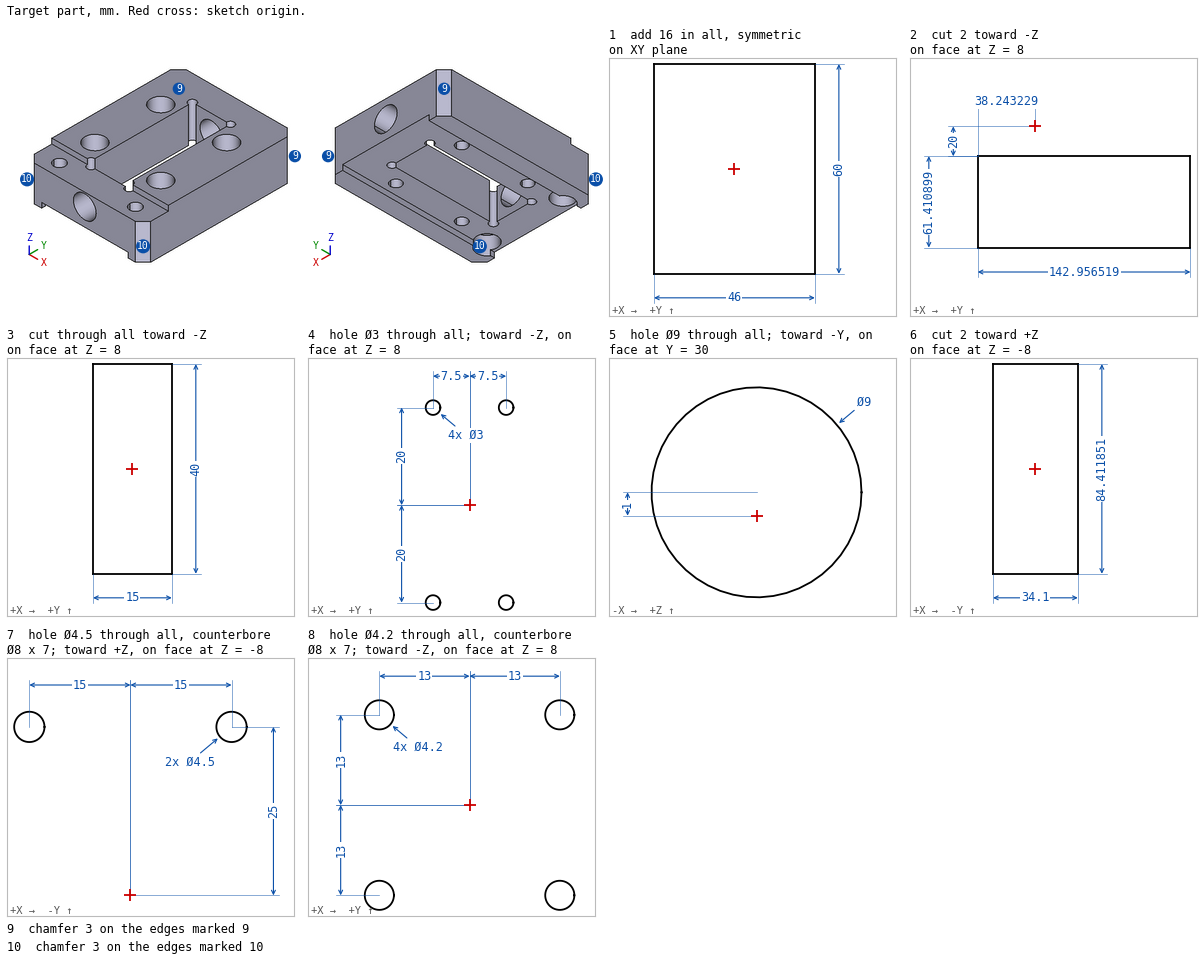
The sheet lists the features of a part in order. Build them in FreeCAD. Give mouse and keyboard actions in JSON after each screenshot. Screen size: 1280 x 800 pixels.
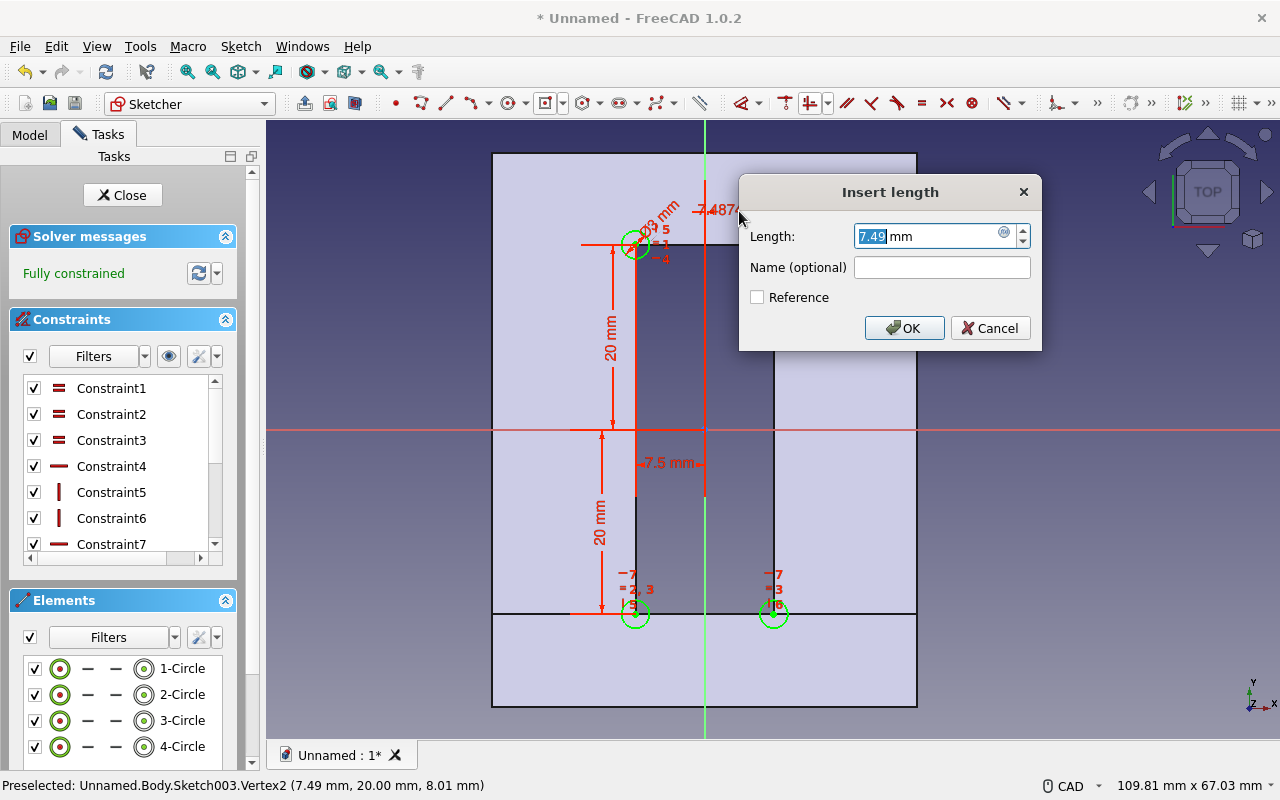
{"action": "type", "text": "7.5"}
{"action": "key", "text": "Return"}
{"action": "key", "text": "Escape"}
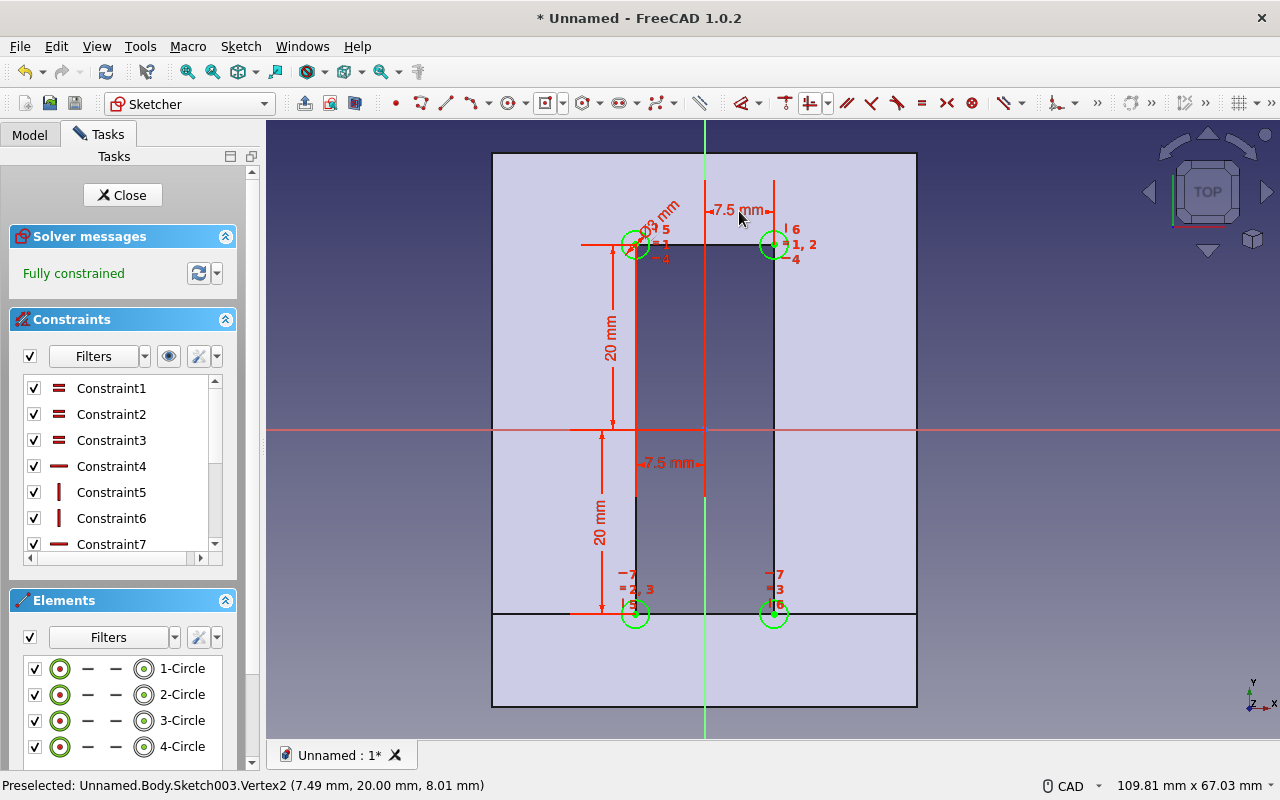
{"action": "left_click", "coordinate": [123, 195]}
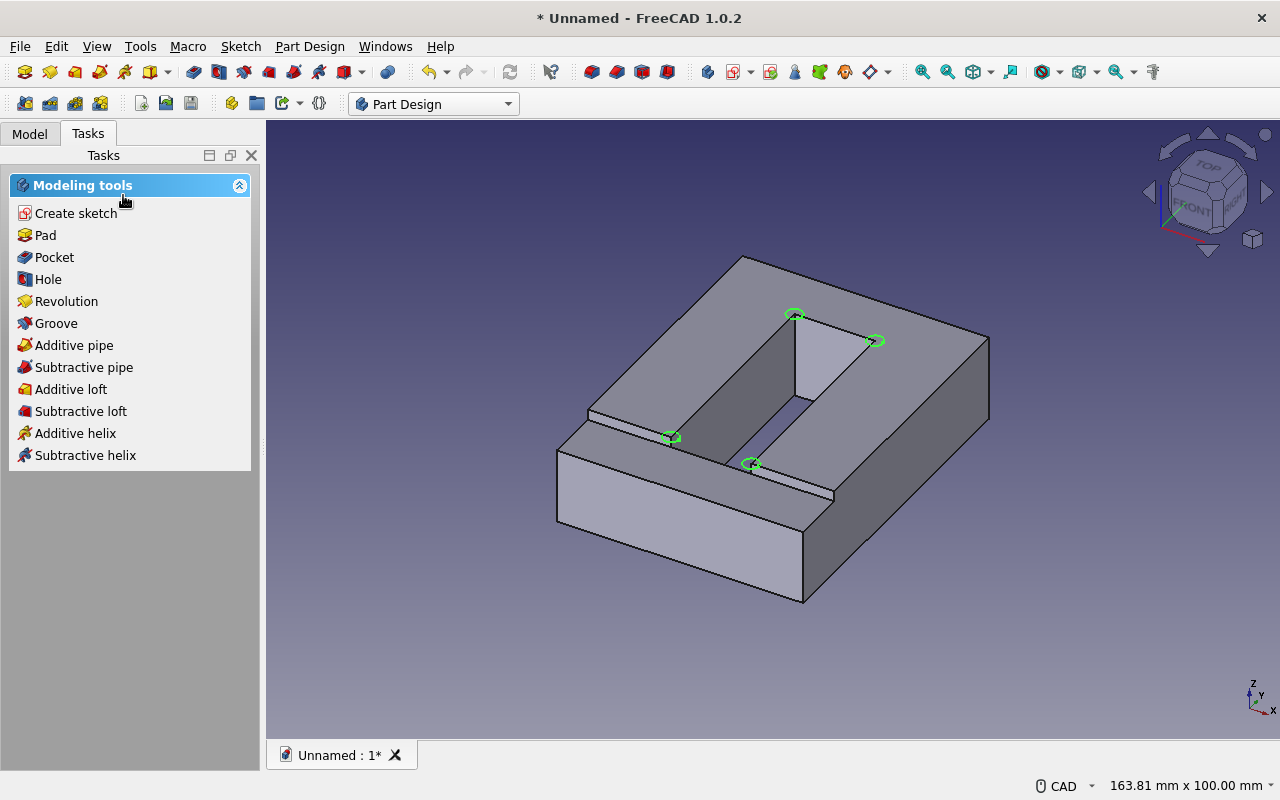
{"action": "left_click", "coordinate": [219, 72]}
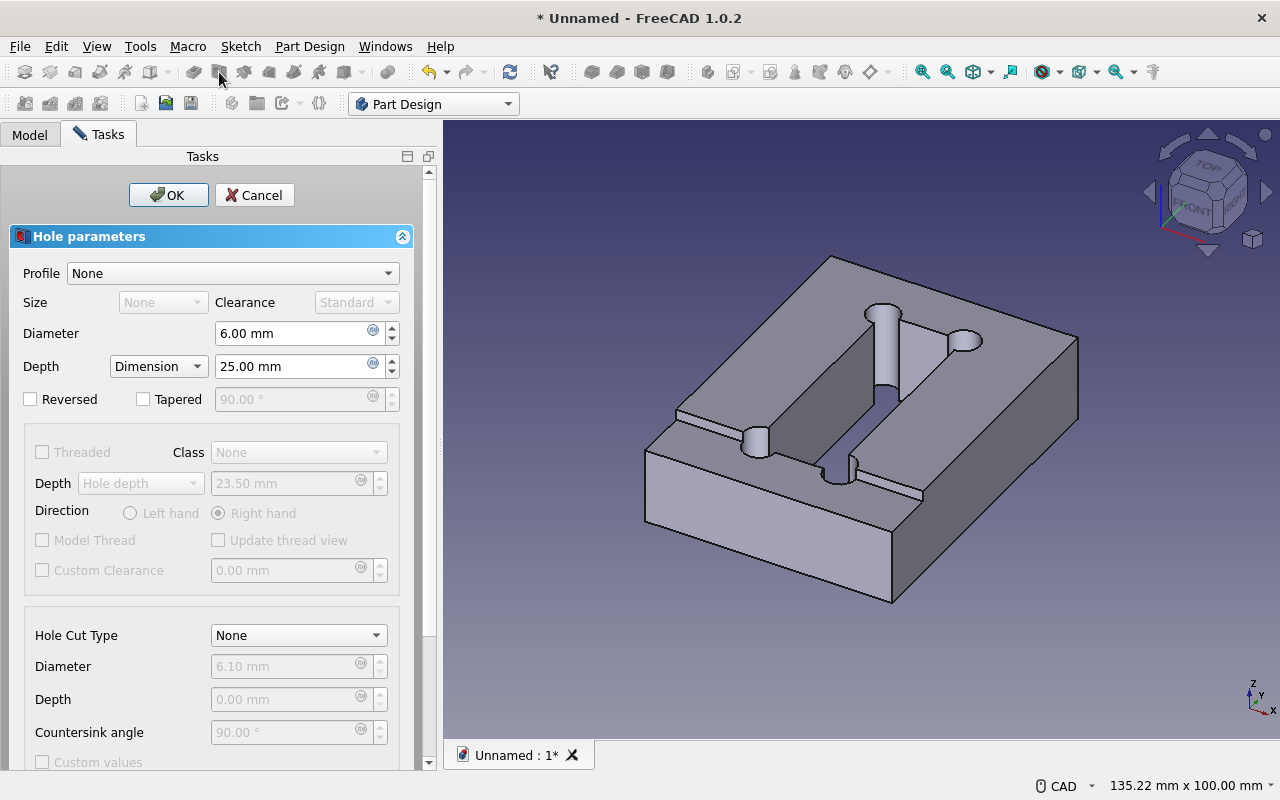
{"action": "triple_click", "coordinate": [300, 334]}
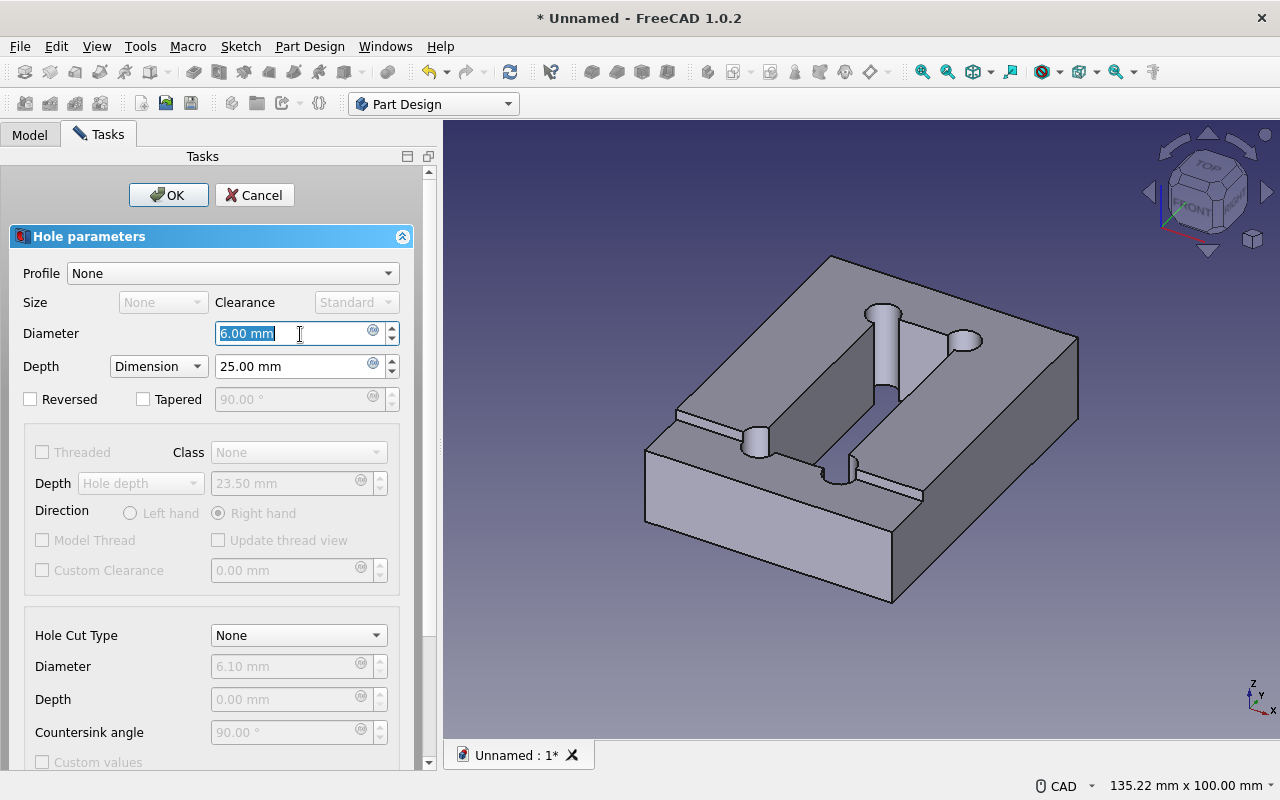
{"action": "type", "text": "3"}
{"action": "key", "text": "Tab"}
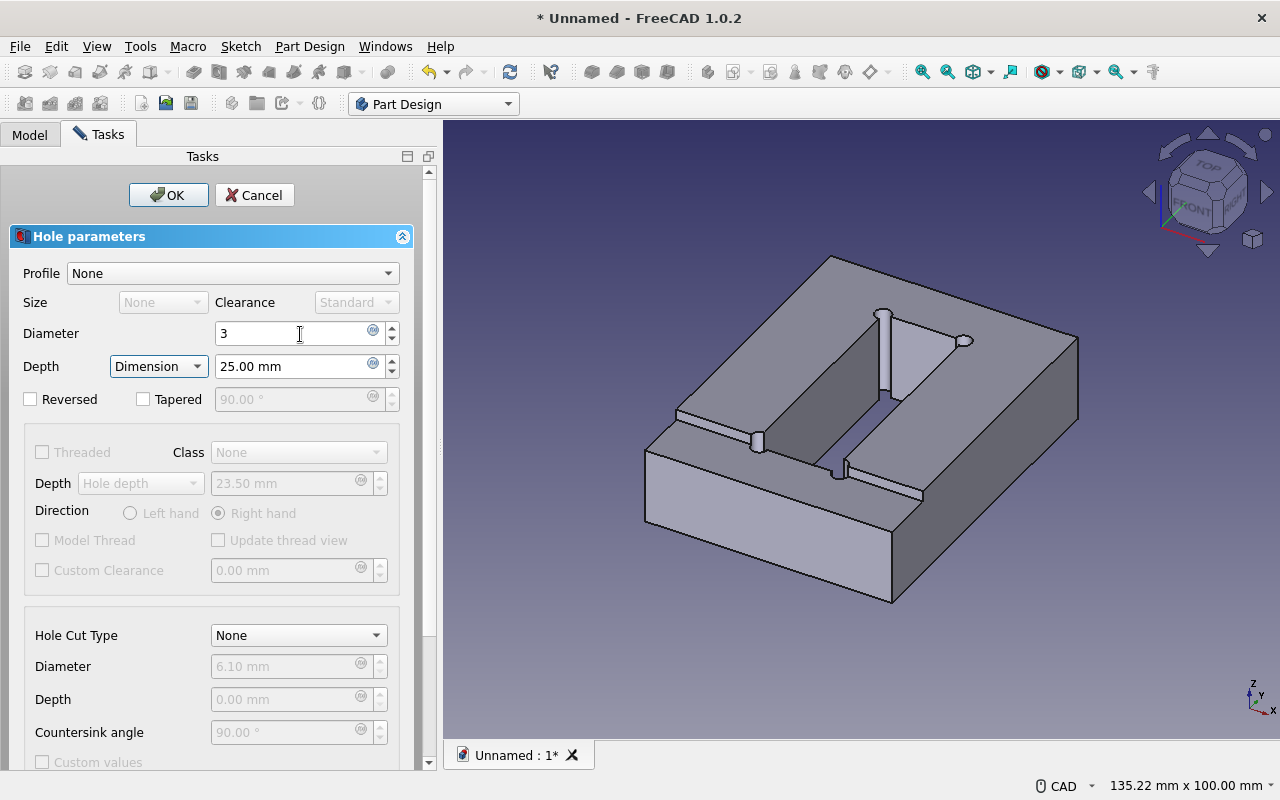
{"action": "left_click", "coordinate": [160, 366]}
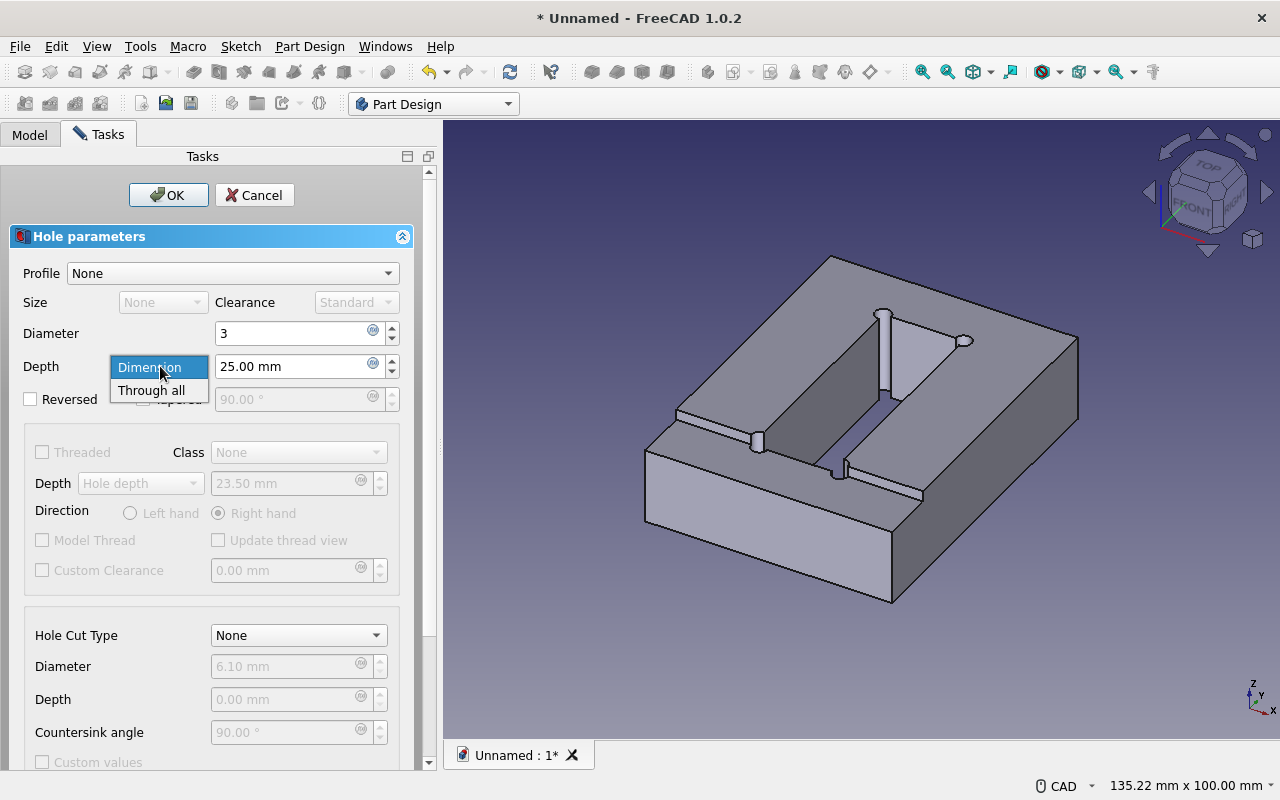
{"action": "left_click", "coordinate": [158, 390]}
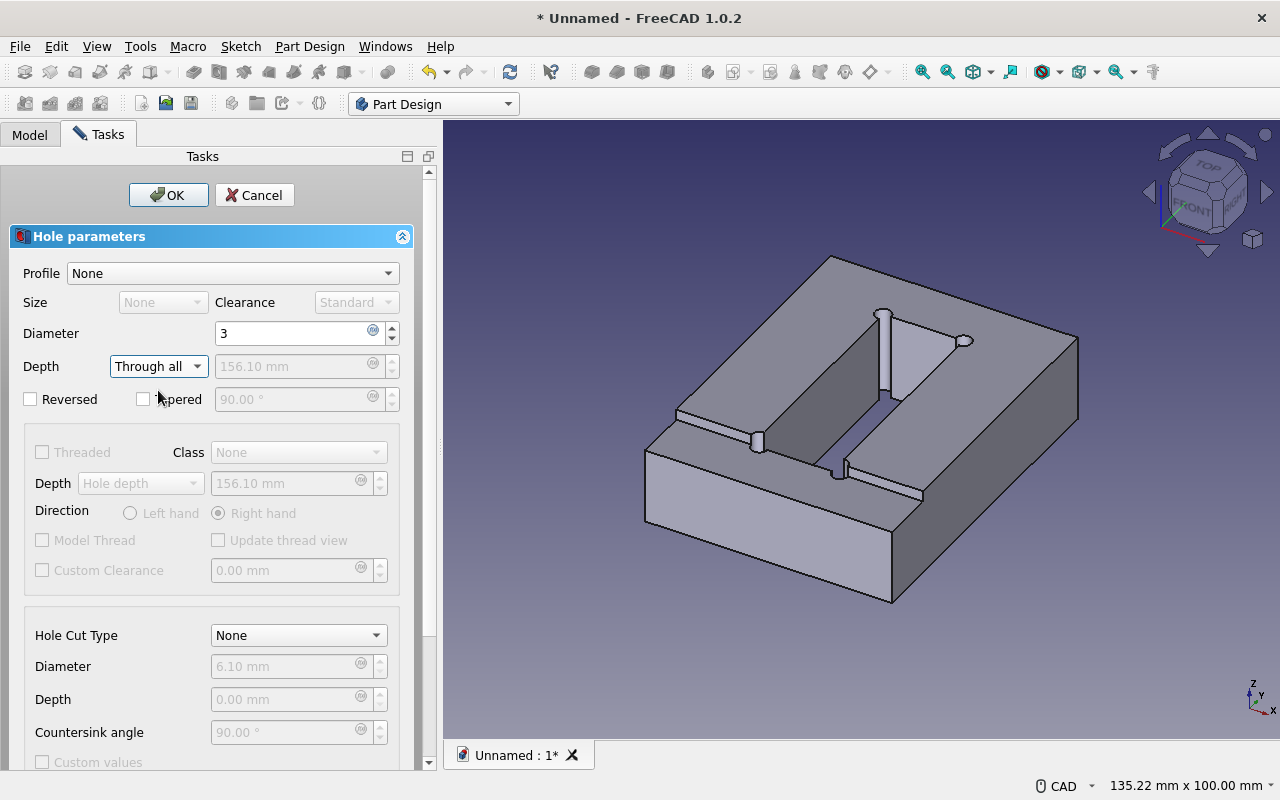
{"action": "left_click", "coordinate": [169, 195]}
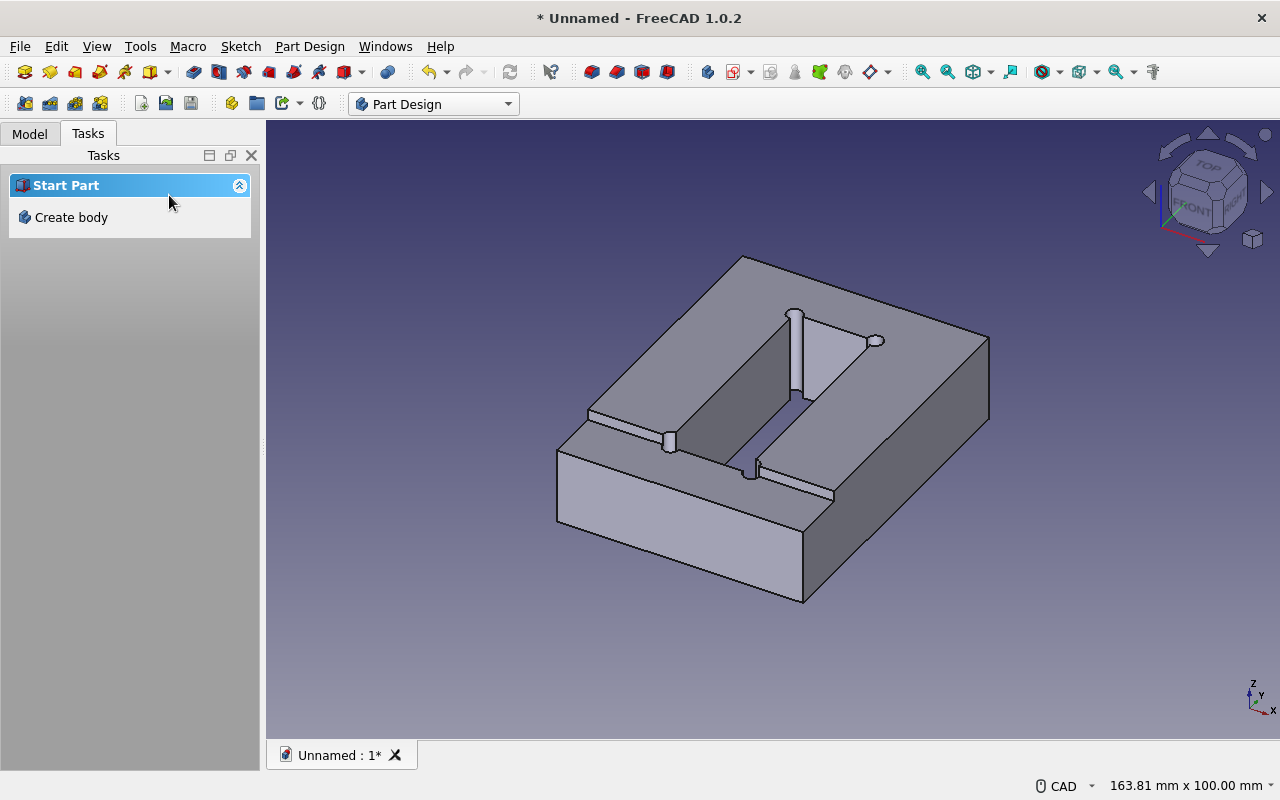
{"action": "key", "text": "4"}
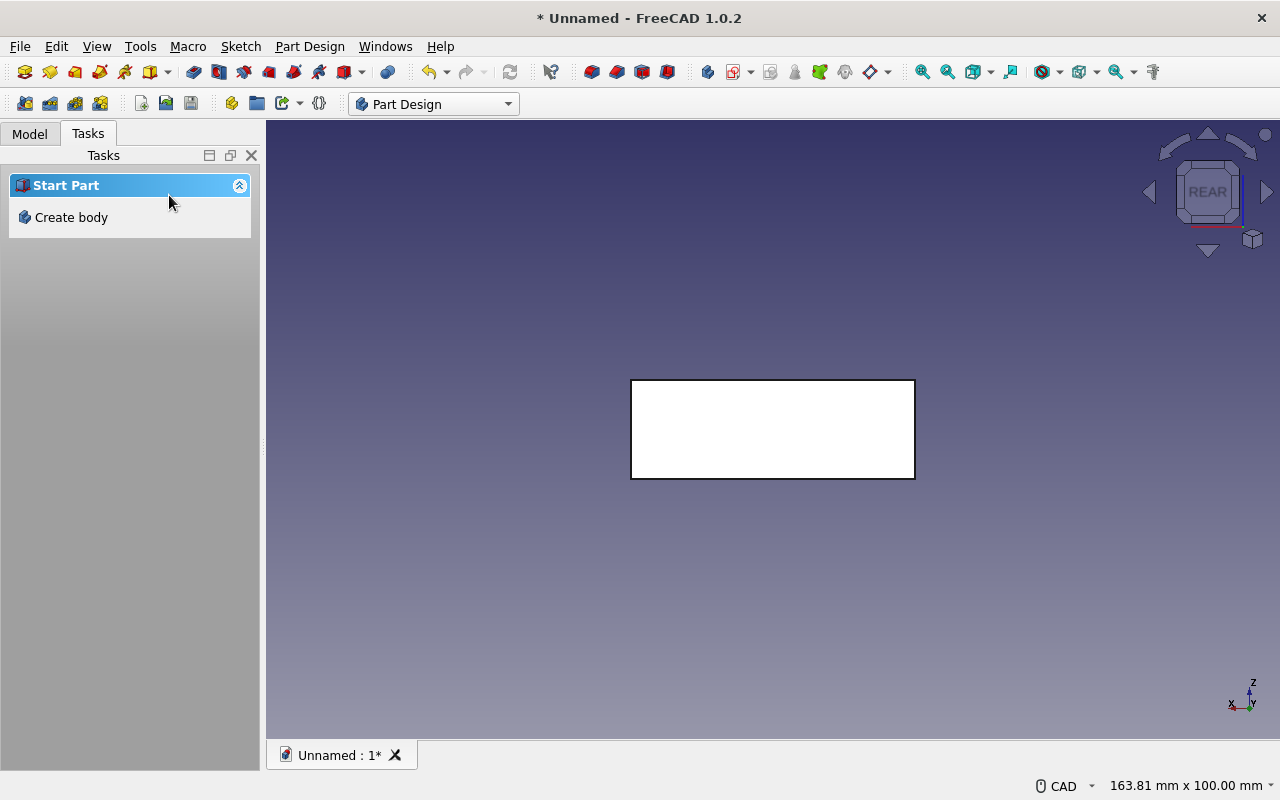
{"action": "left_click", "coordinate": [923, 72]}